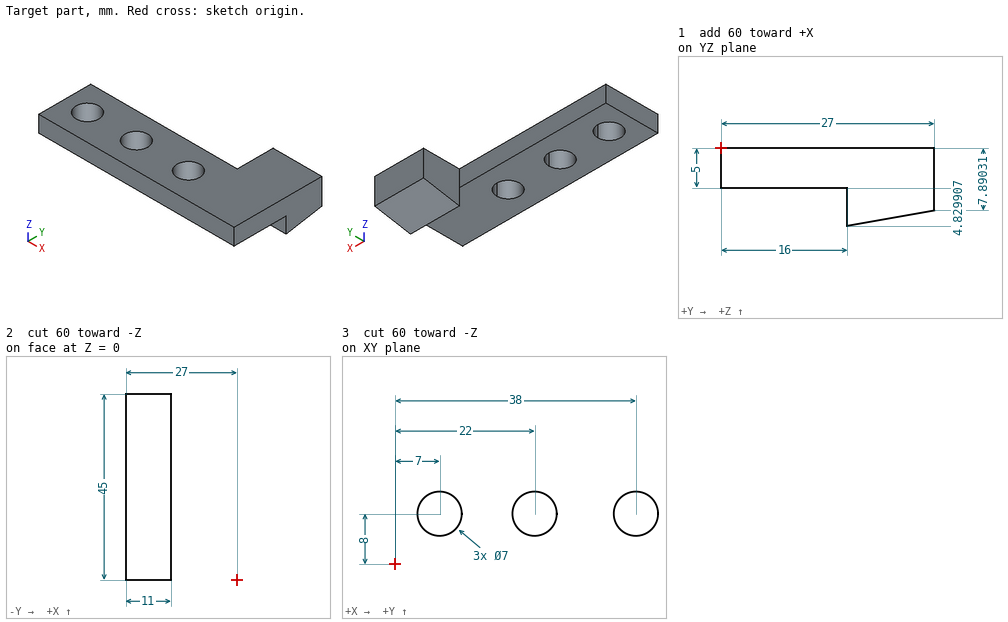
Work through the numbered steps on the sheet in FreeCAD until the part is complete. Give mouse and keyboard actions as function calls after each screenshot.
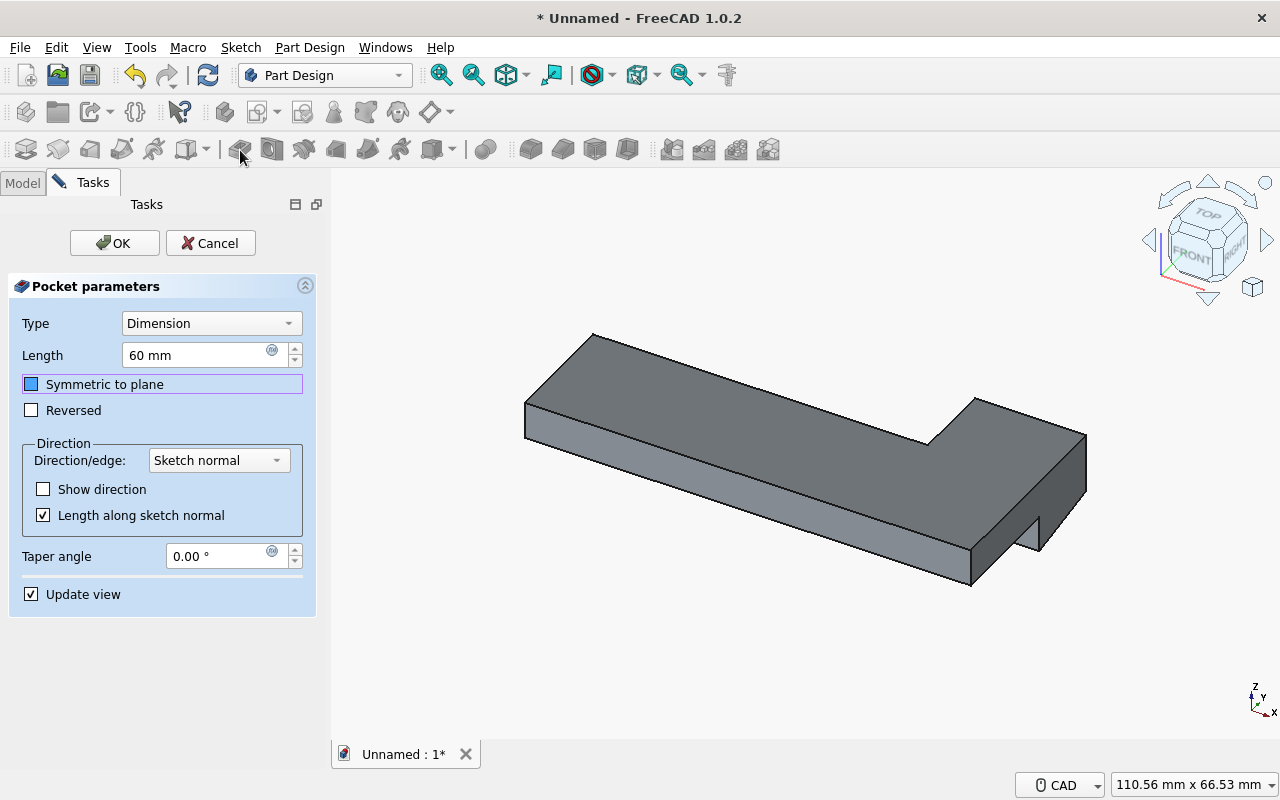
click(115, 243)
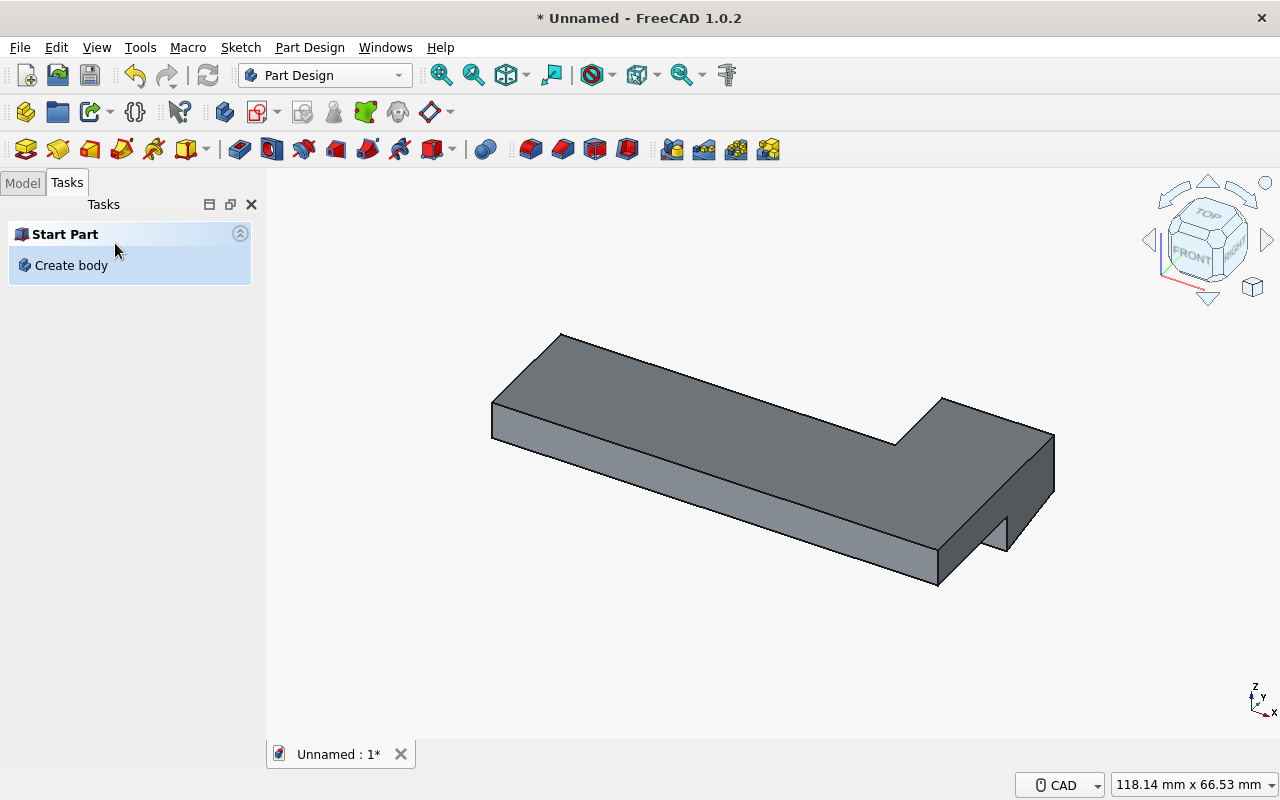
click(258, 112)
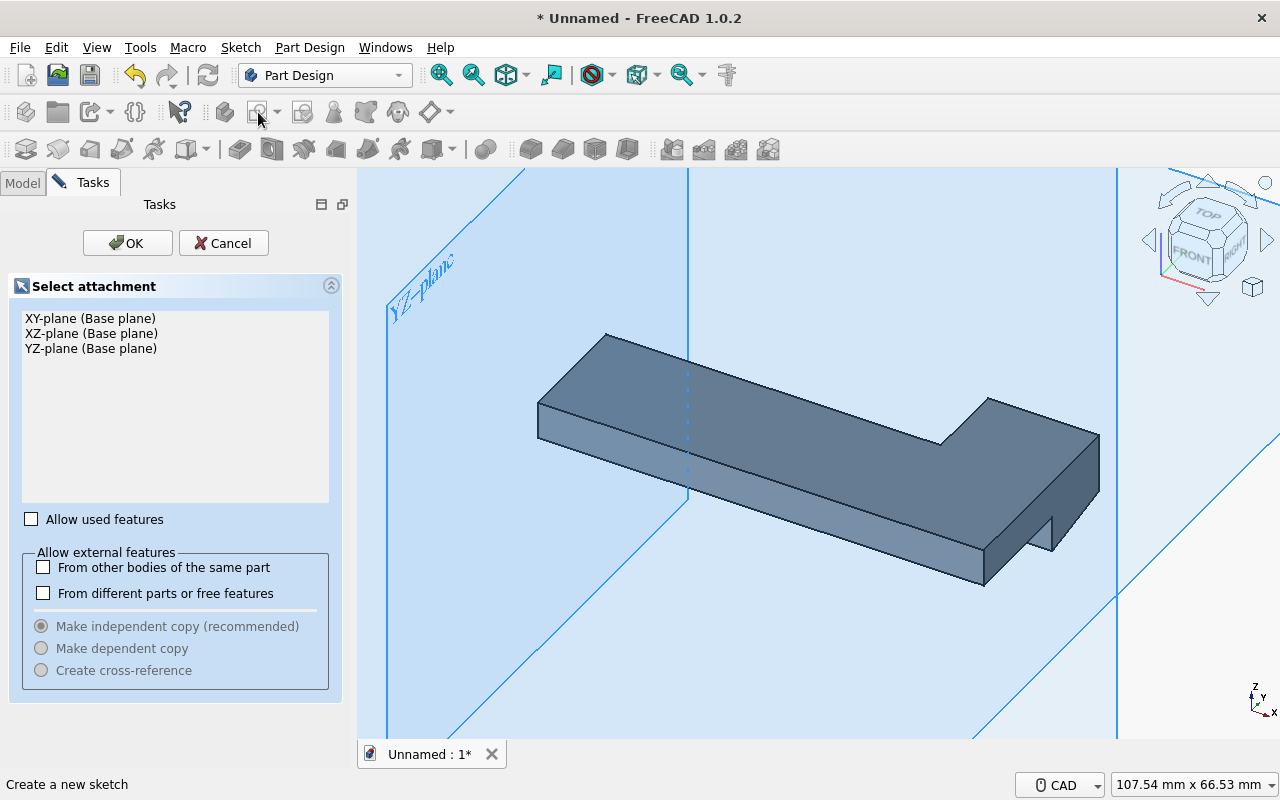
click(82, 318)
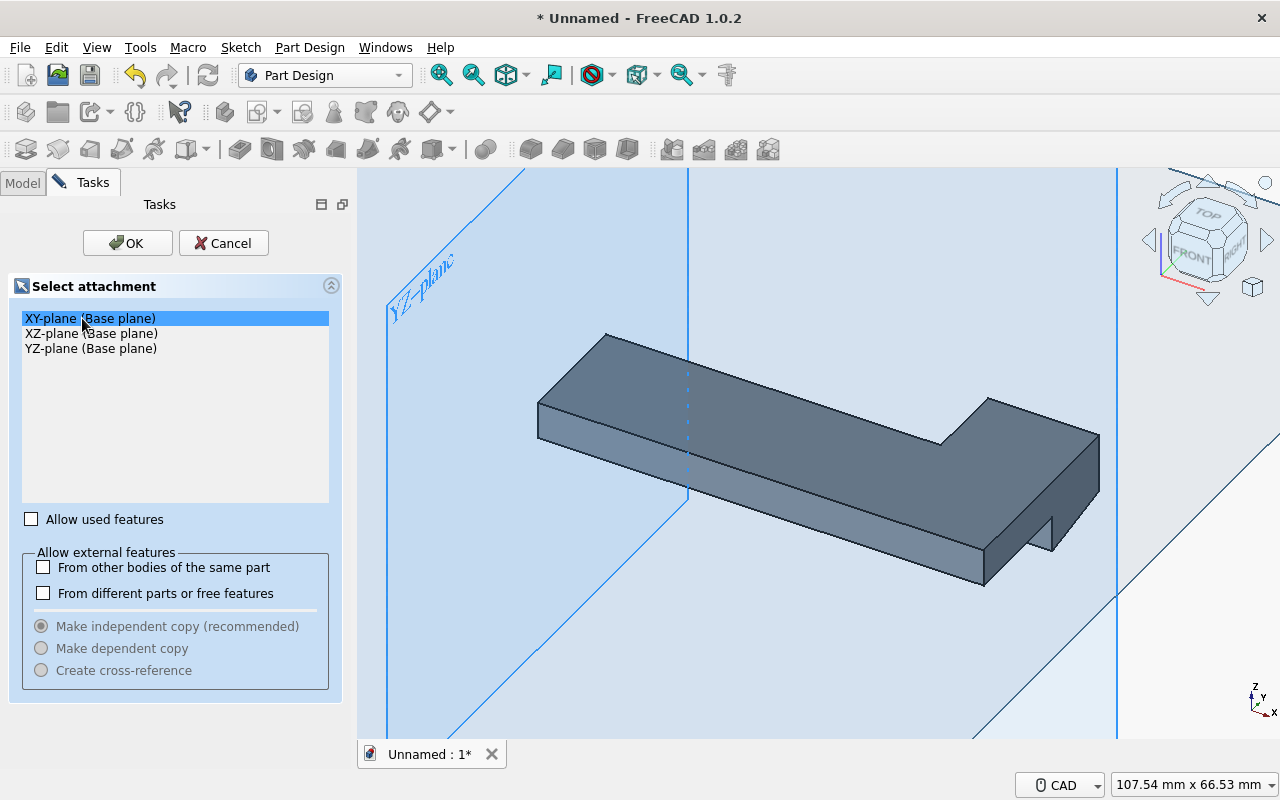
click(128, 243)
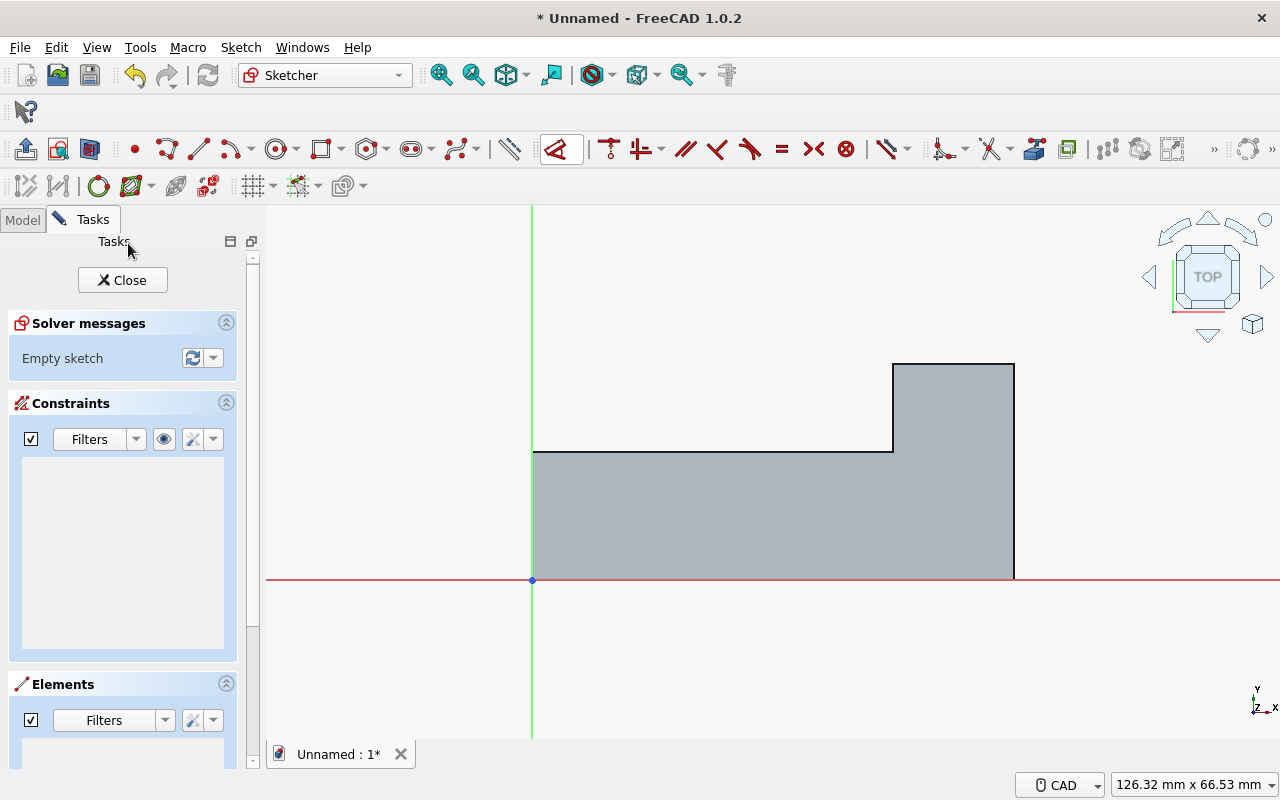
scroll(692, 610, up, 3)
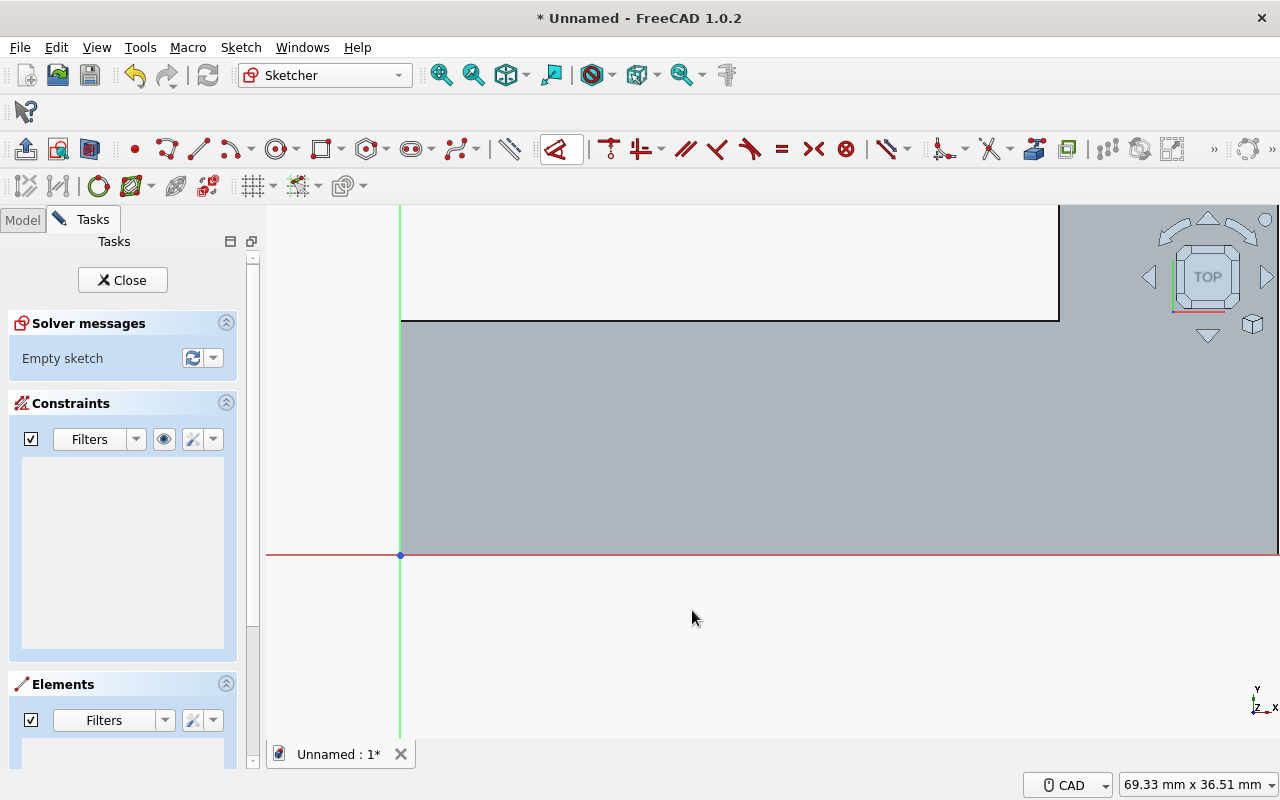
click(276, 150)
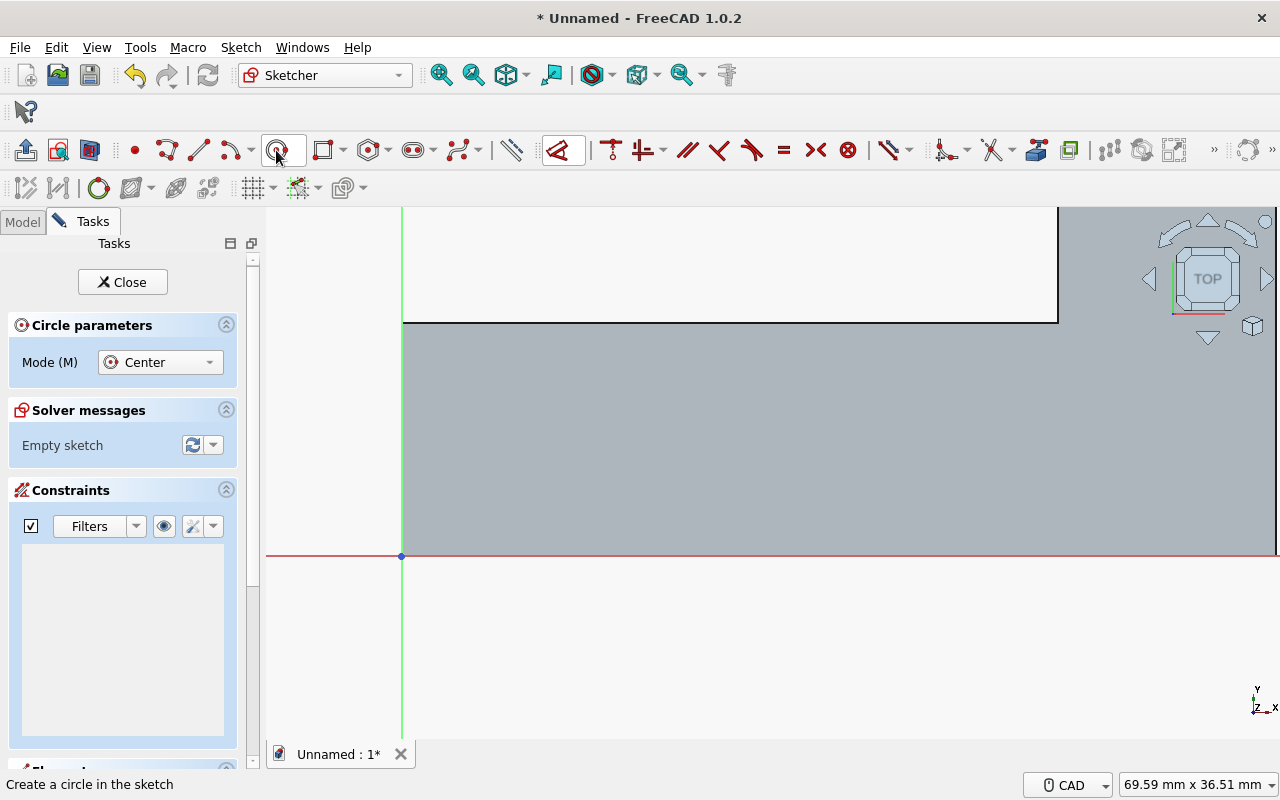
click(504, 439)
move(540, 403)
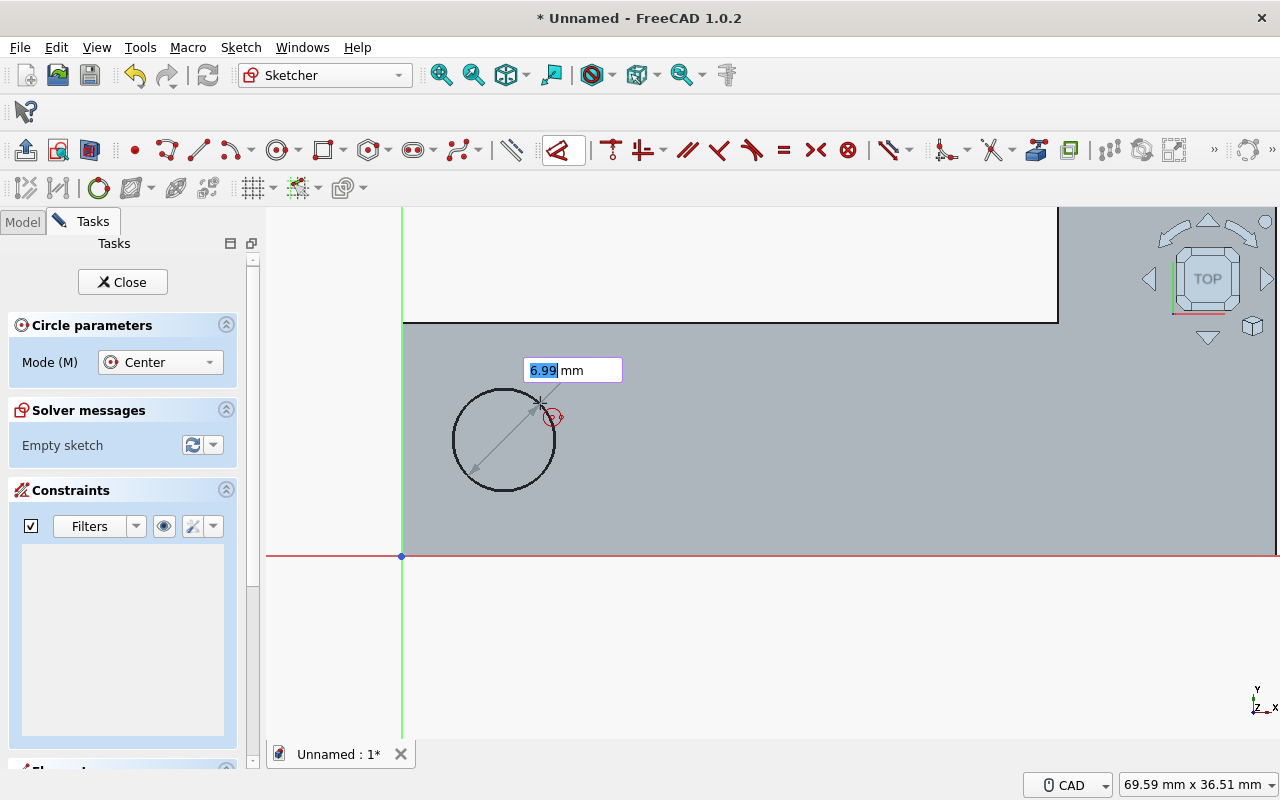
text(7)
key(Return)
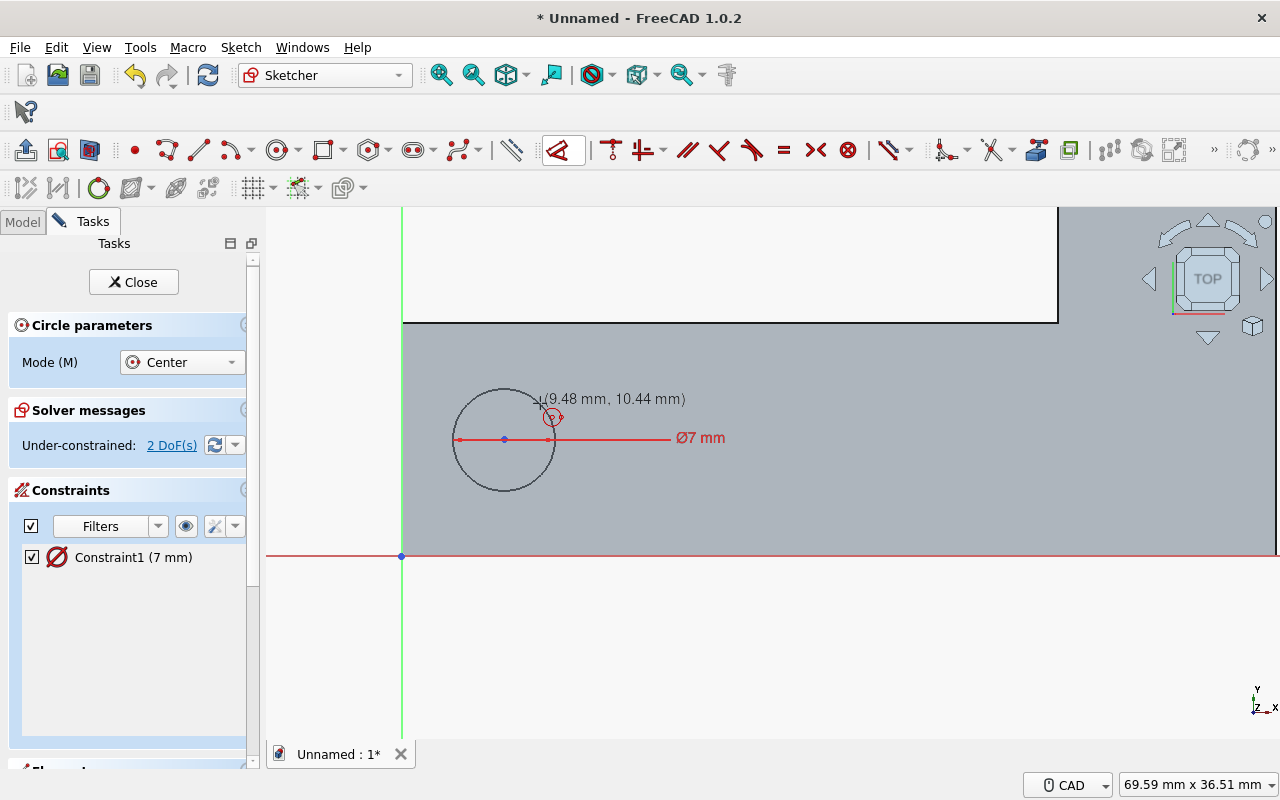
click(722, 439)
move(758, 403)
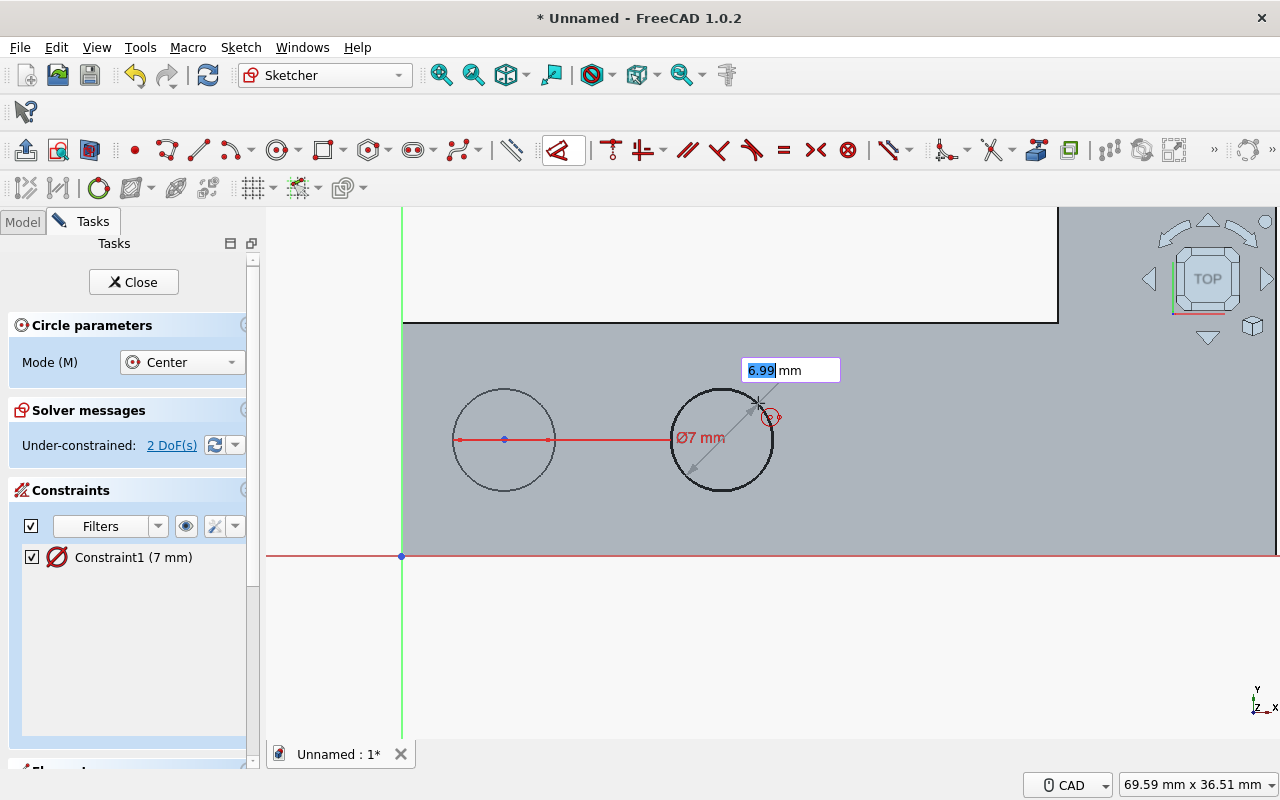
text(7)
key(Return)